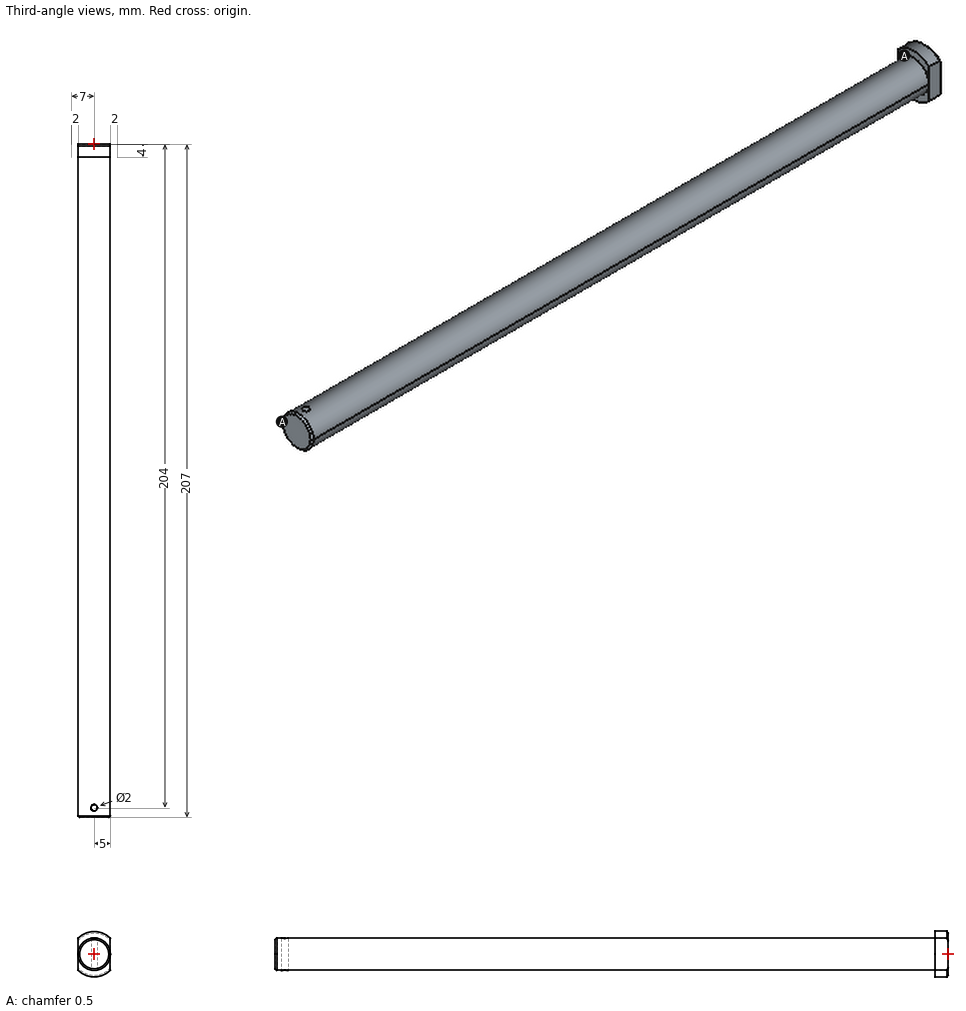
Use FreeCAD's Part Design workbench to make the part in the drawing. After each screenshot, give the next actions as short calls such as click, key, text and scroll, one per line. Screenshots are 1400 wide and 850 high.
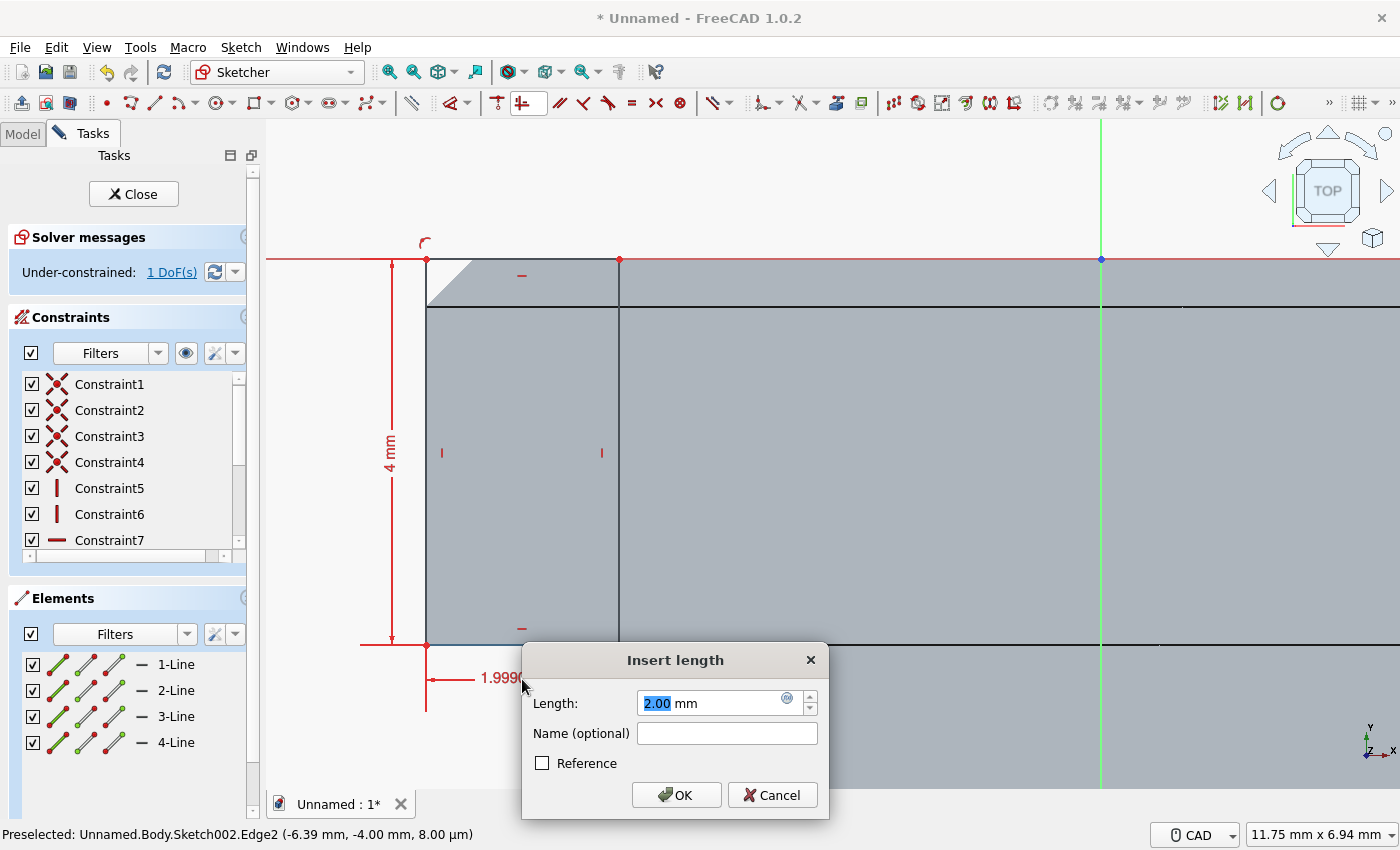
text(2)
key(Return)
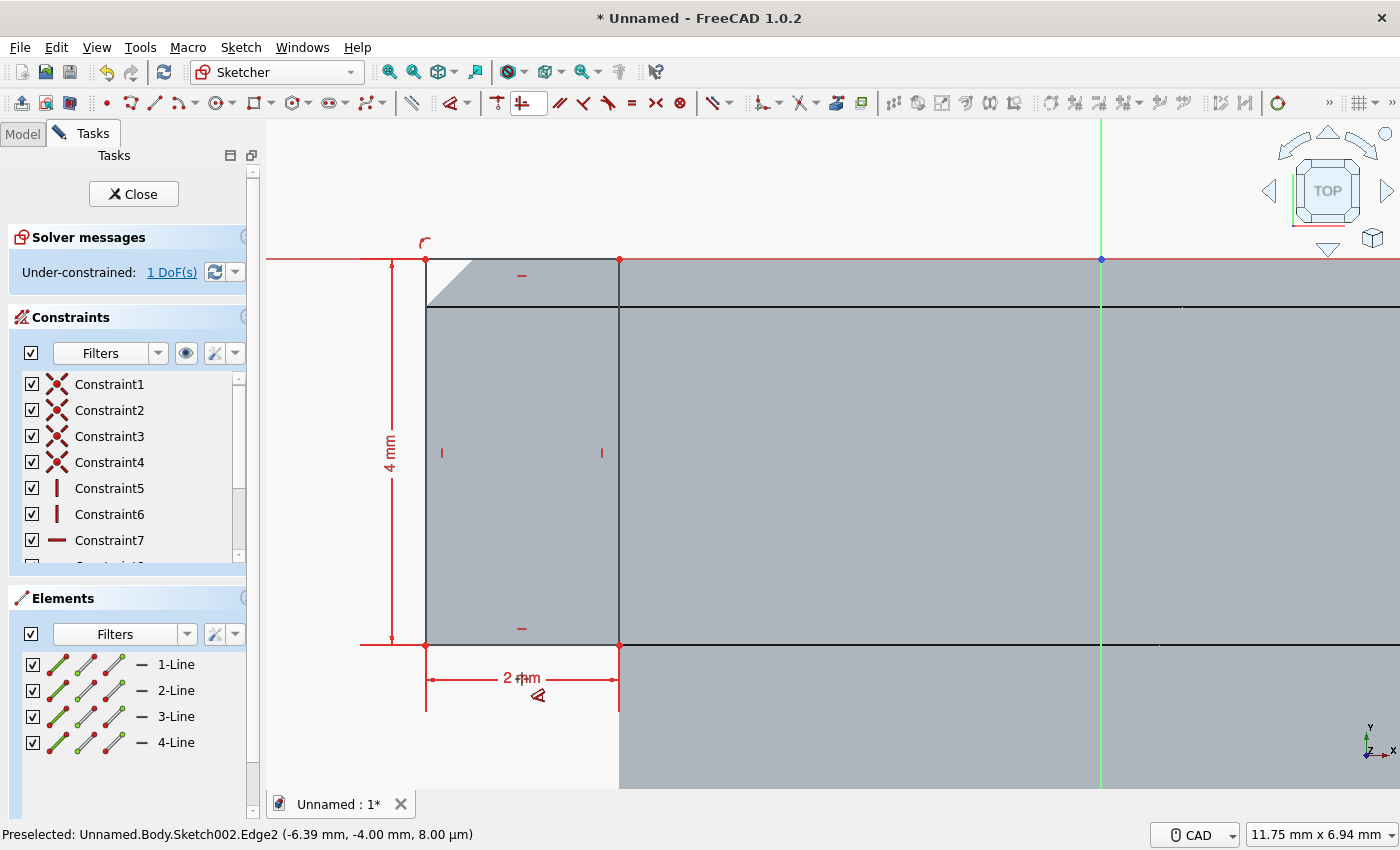
click(426, 259)
click(764, 225)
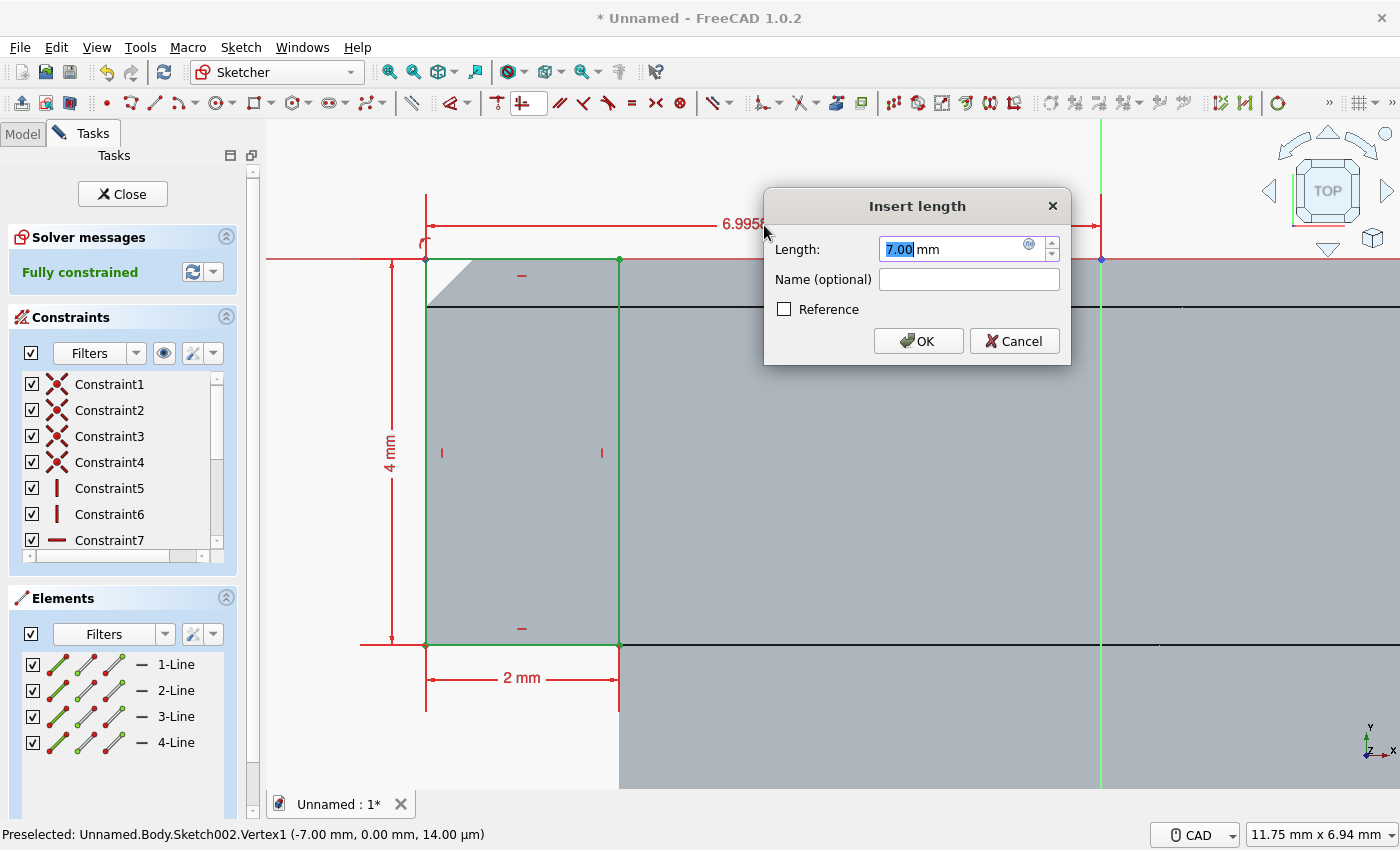
text(7)
key(Return)
key(Escape)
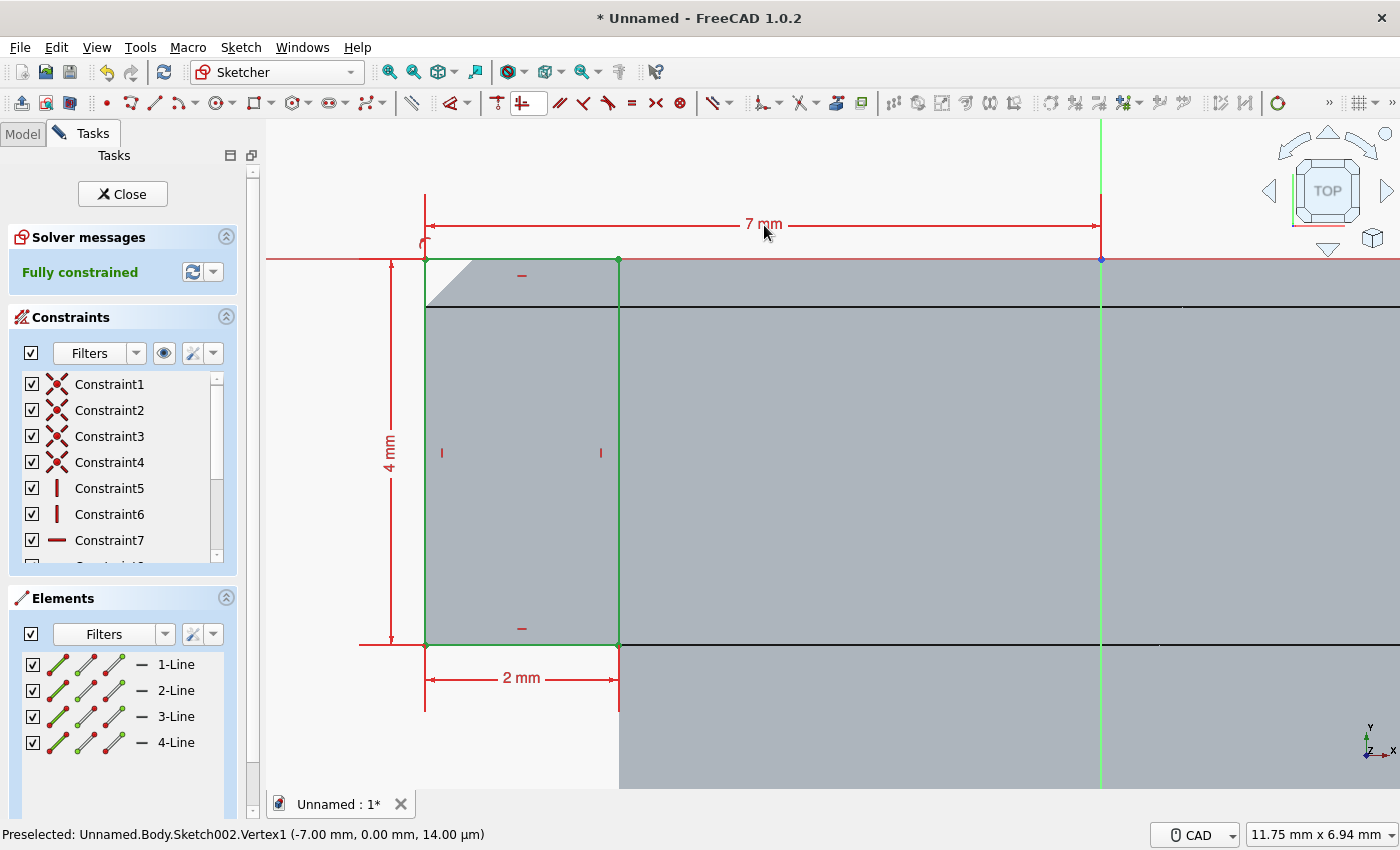
click(123, 194)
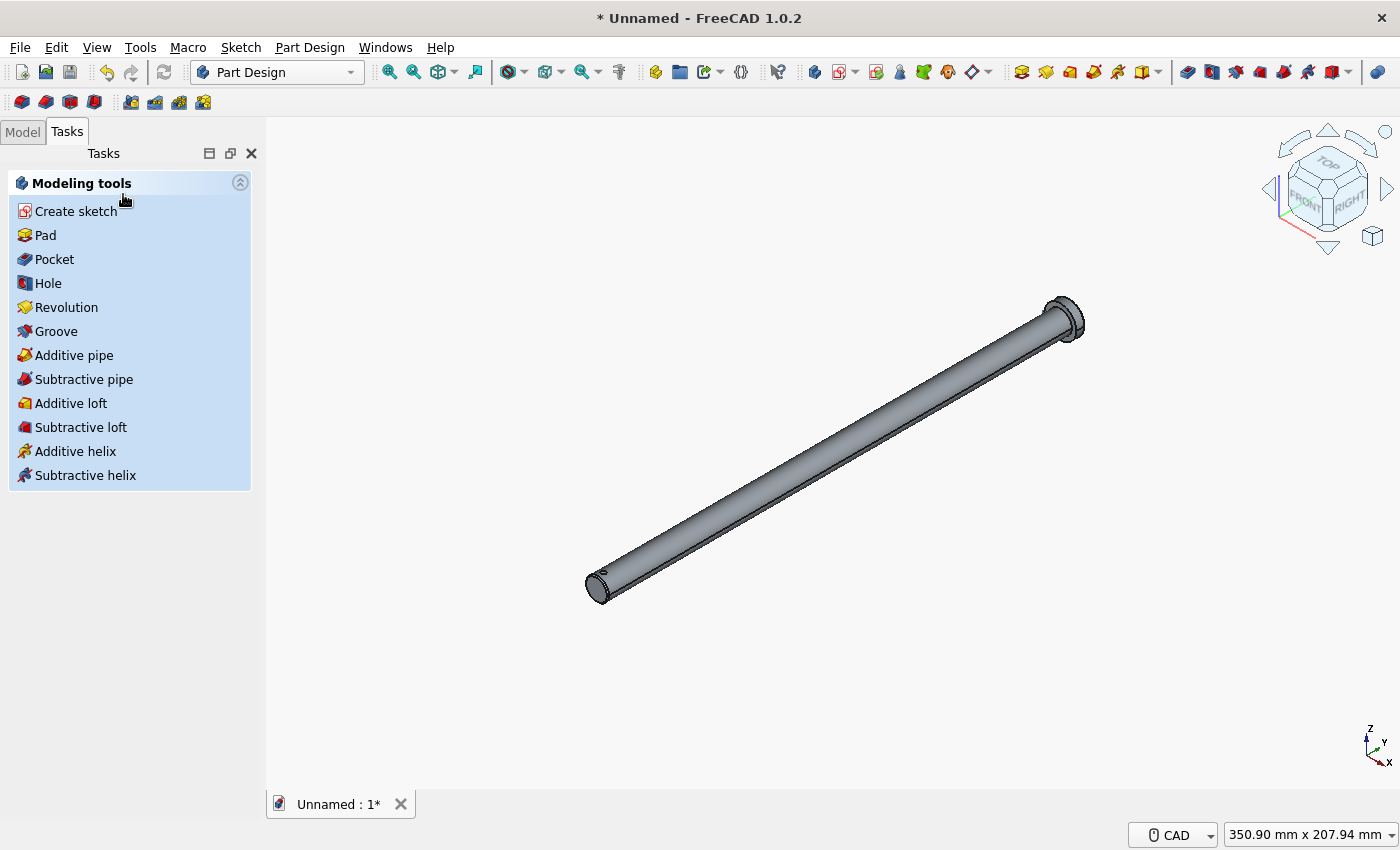
click(1188, 72)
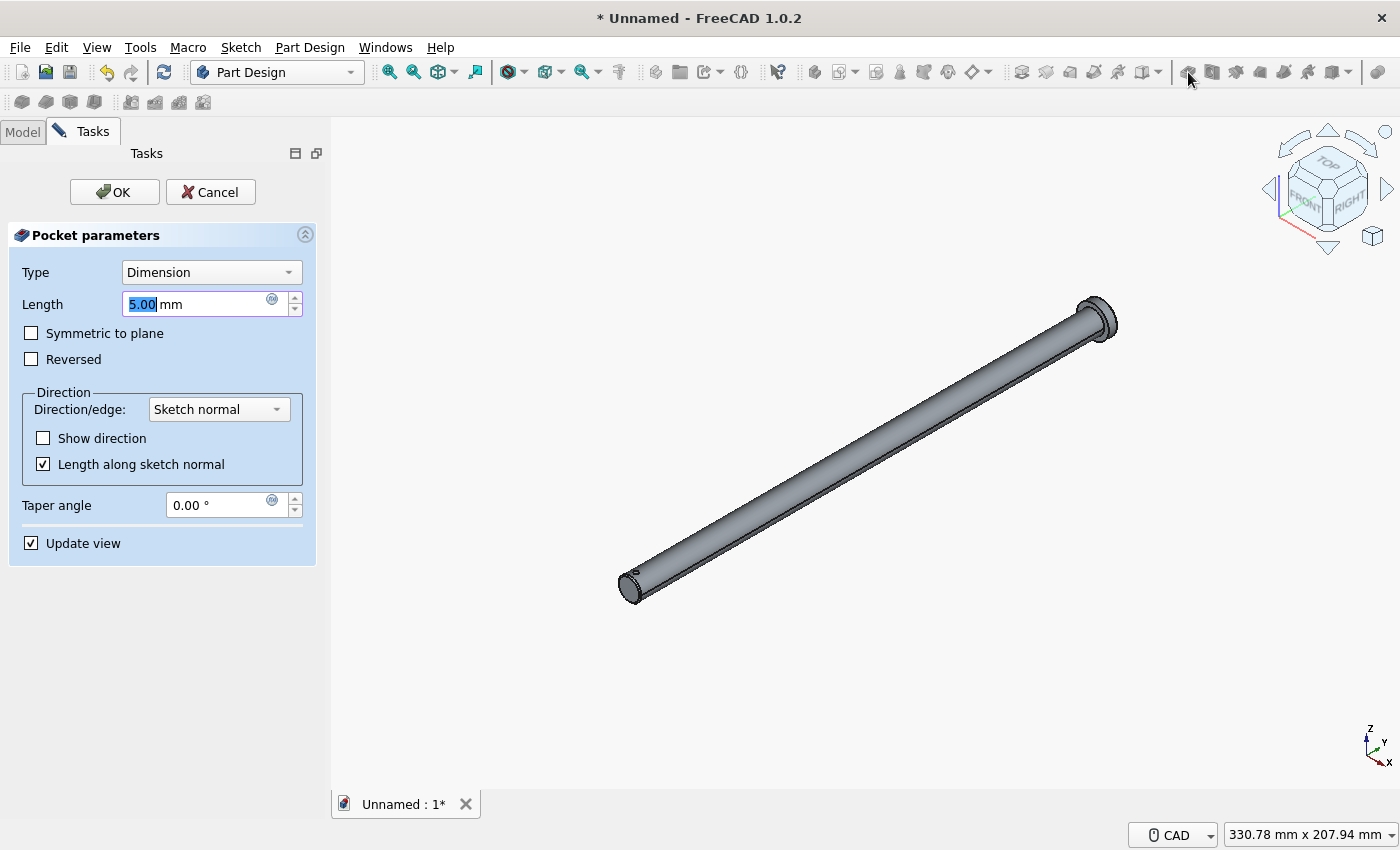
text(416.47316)
key(Tab)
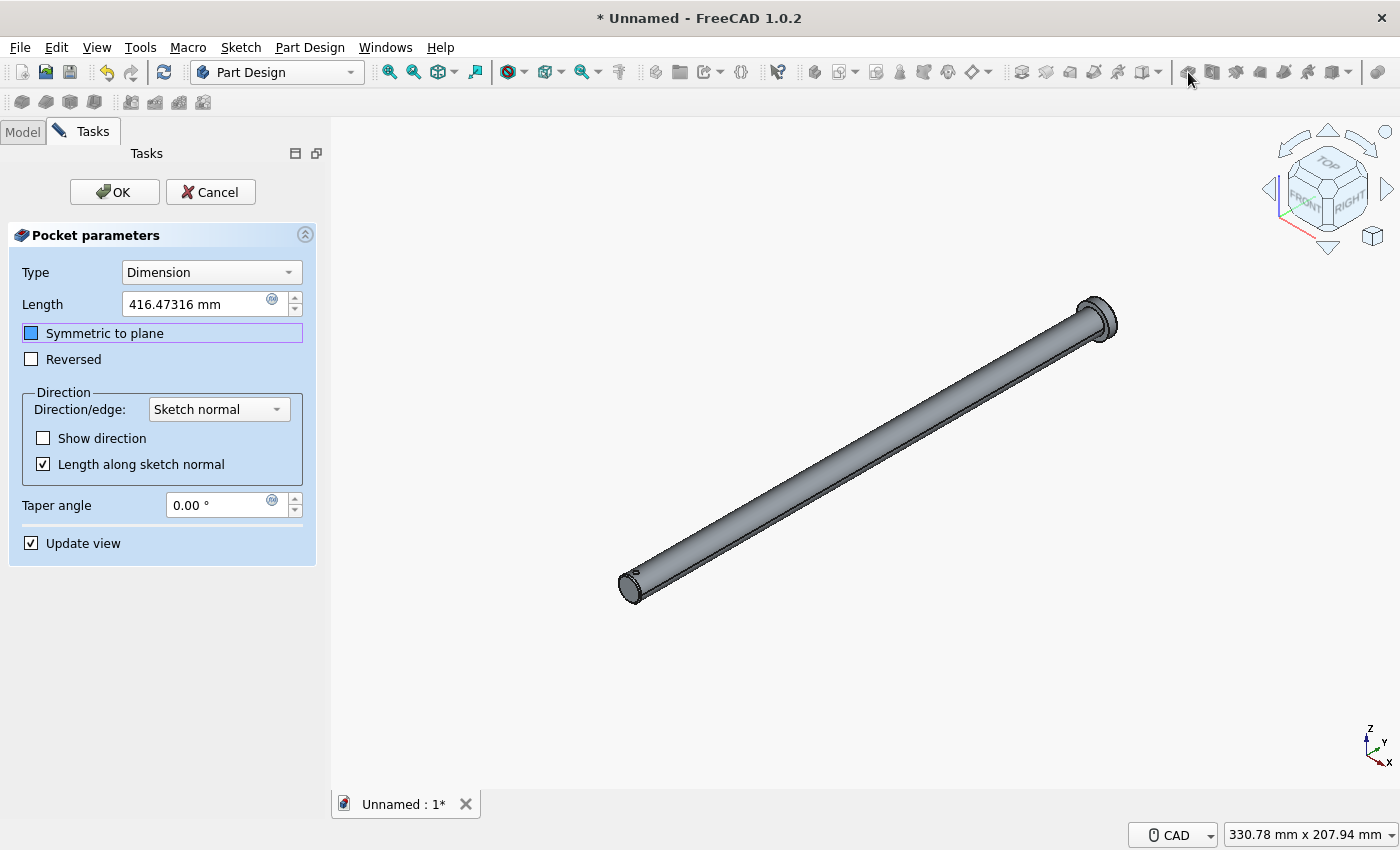
click(30, 333)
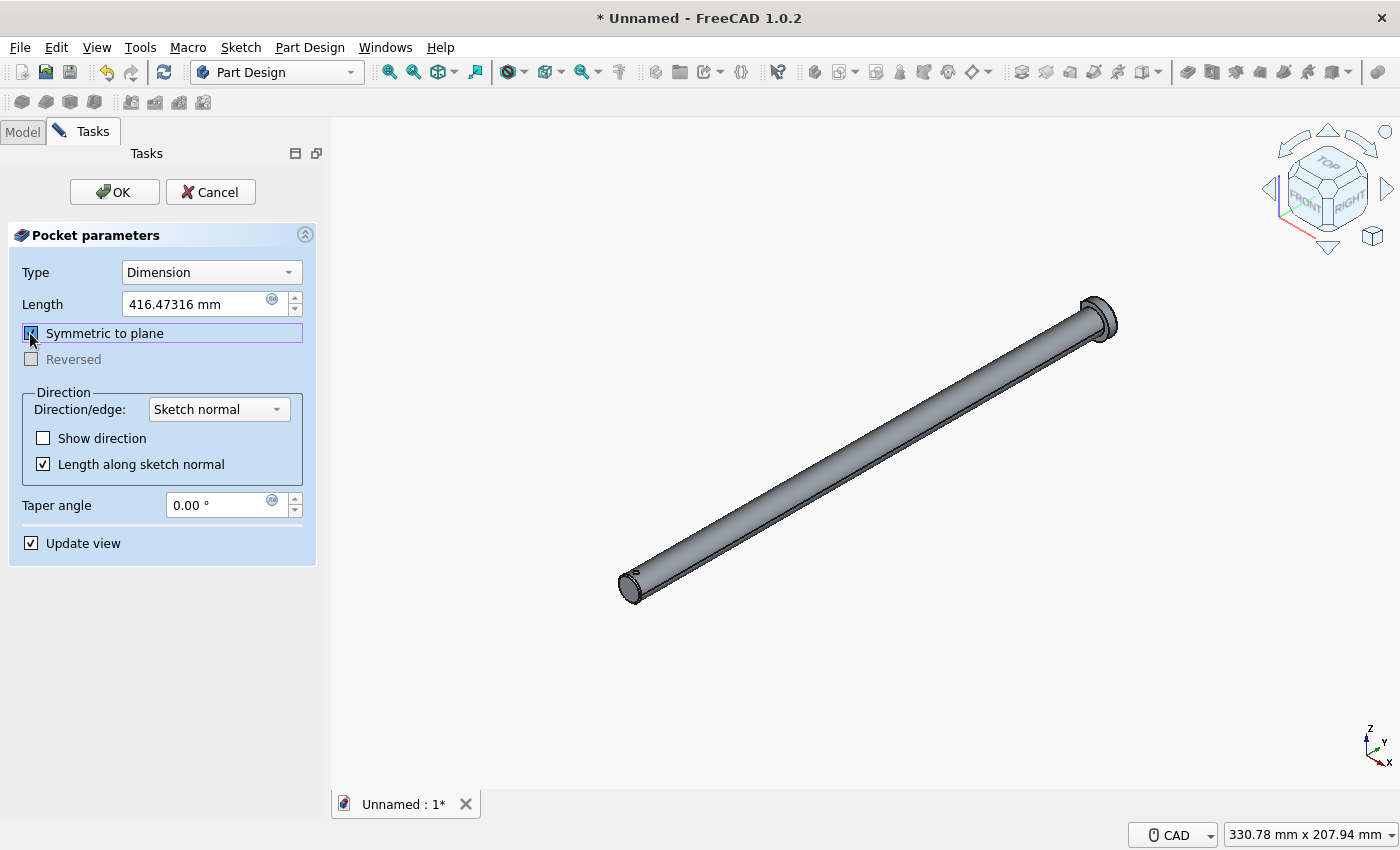
click(115, 192)